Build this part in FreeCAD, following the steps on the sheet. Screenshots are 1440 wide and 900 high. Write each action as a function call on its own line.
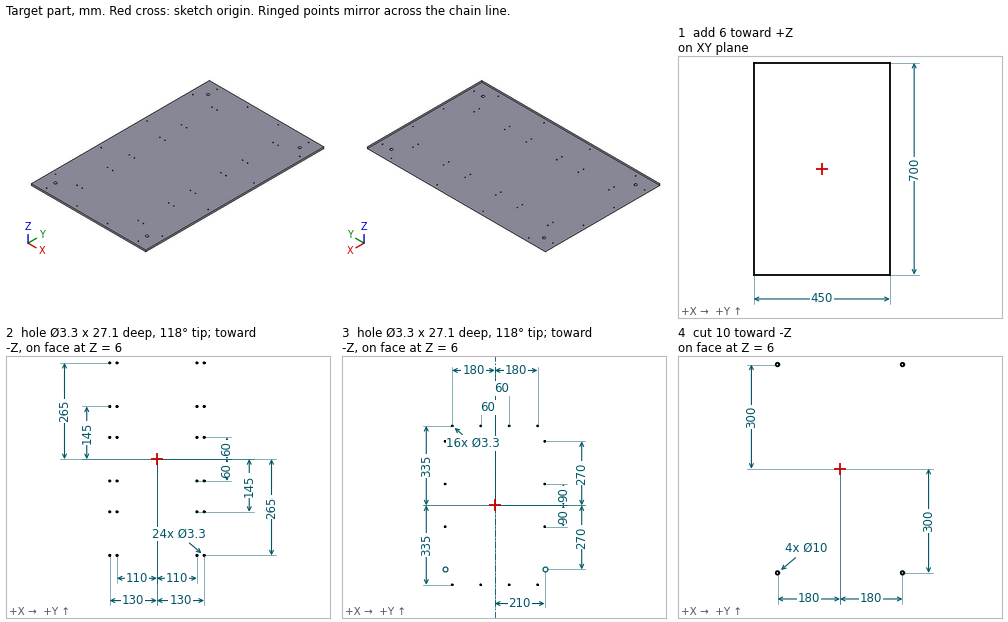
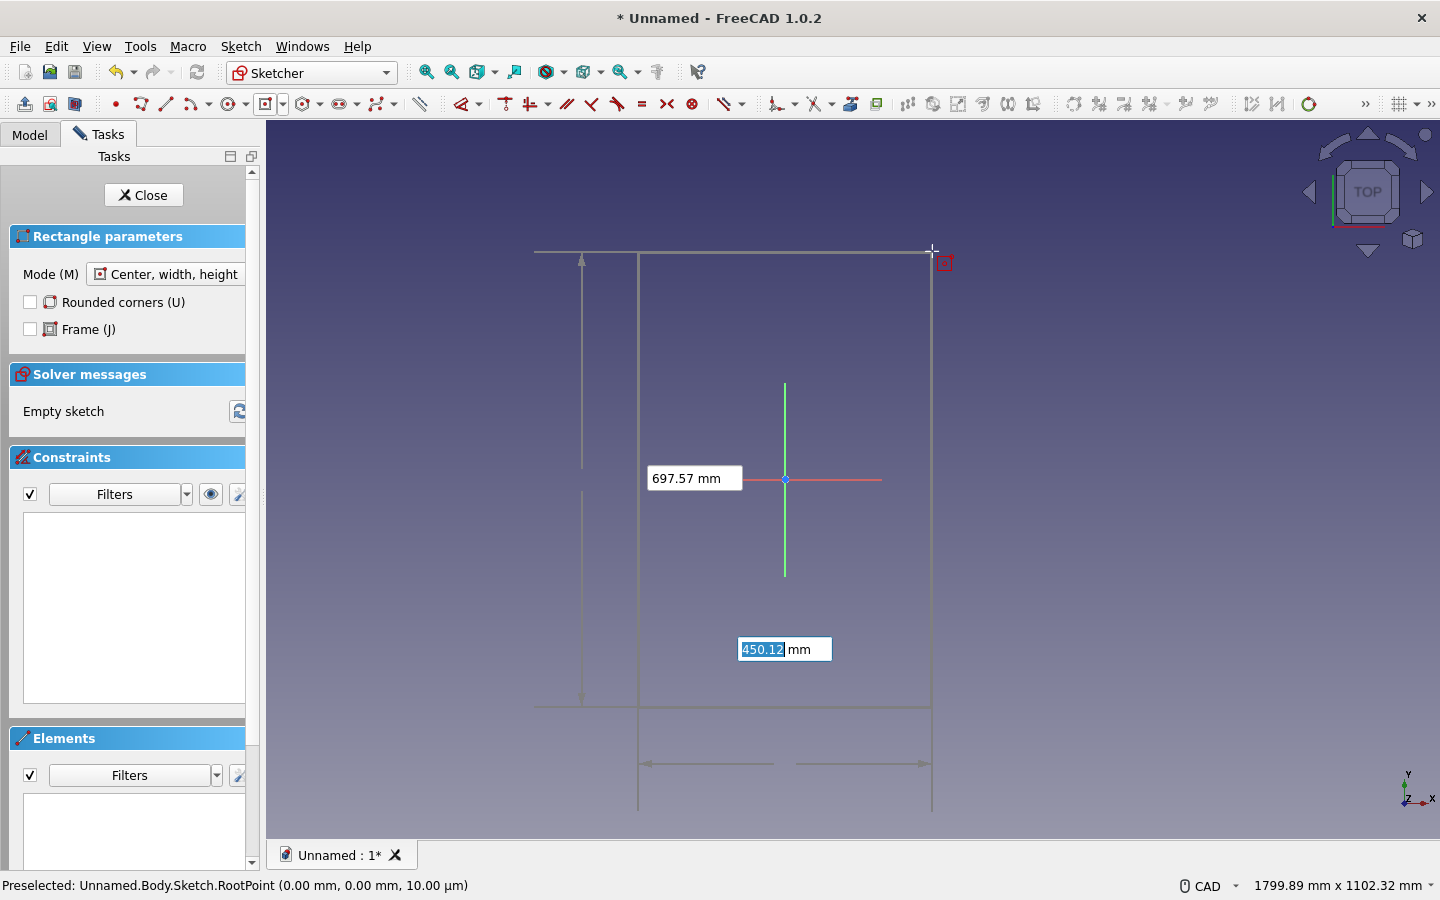
text(450)
key(Tab)
text(700)
key(Return)
key(Escape)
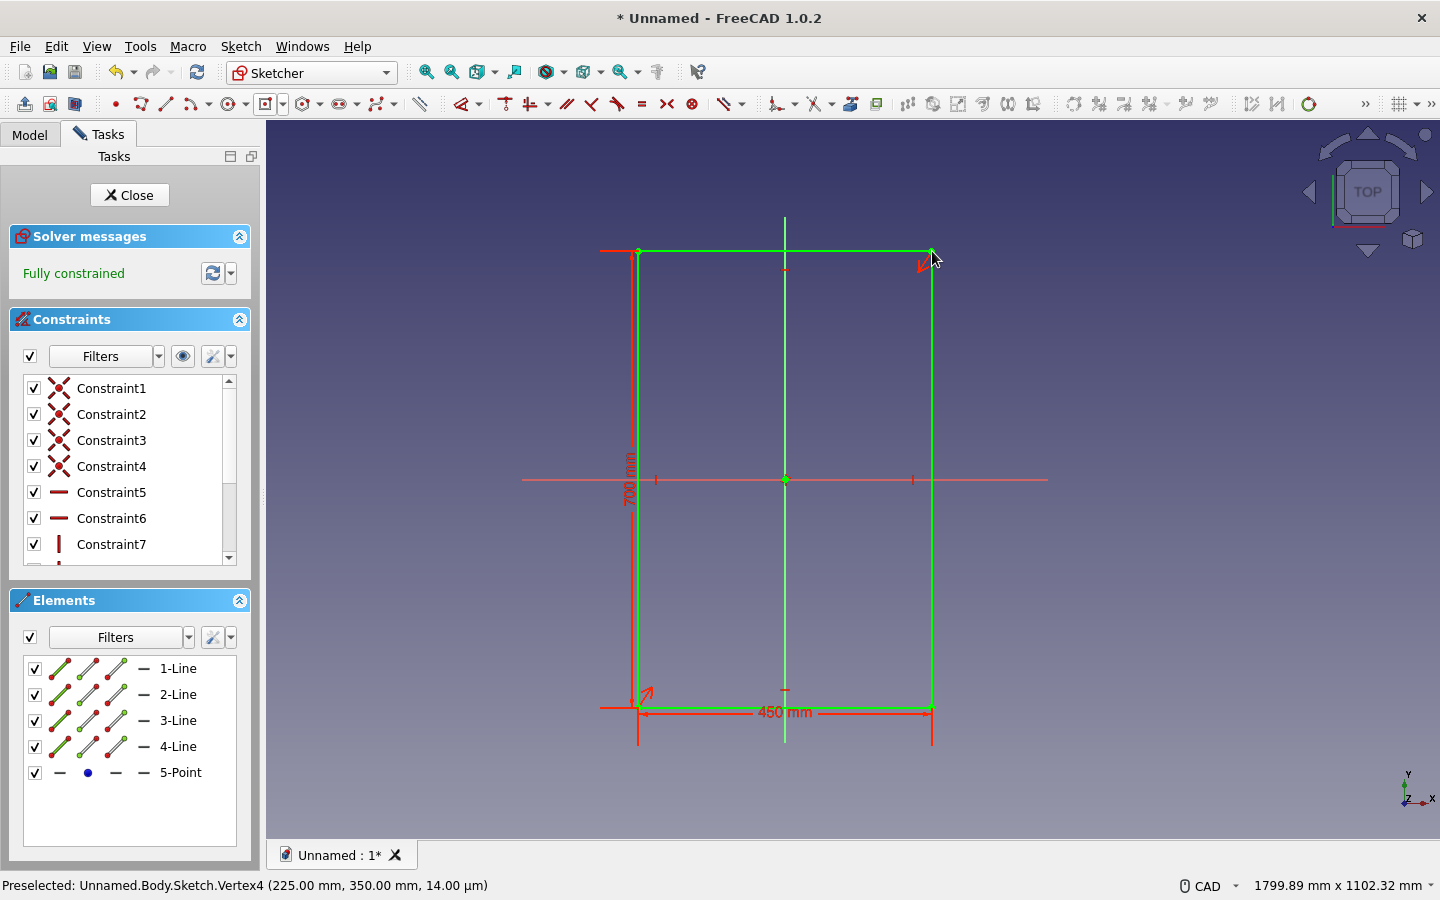
click(130, 195)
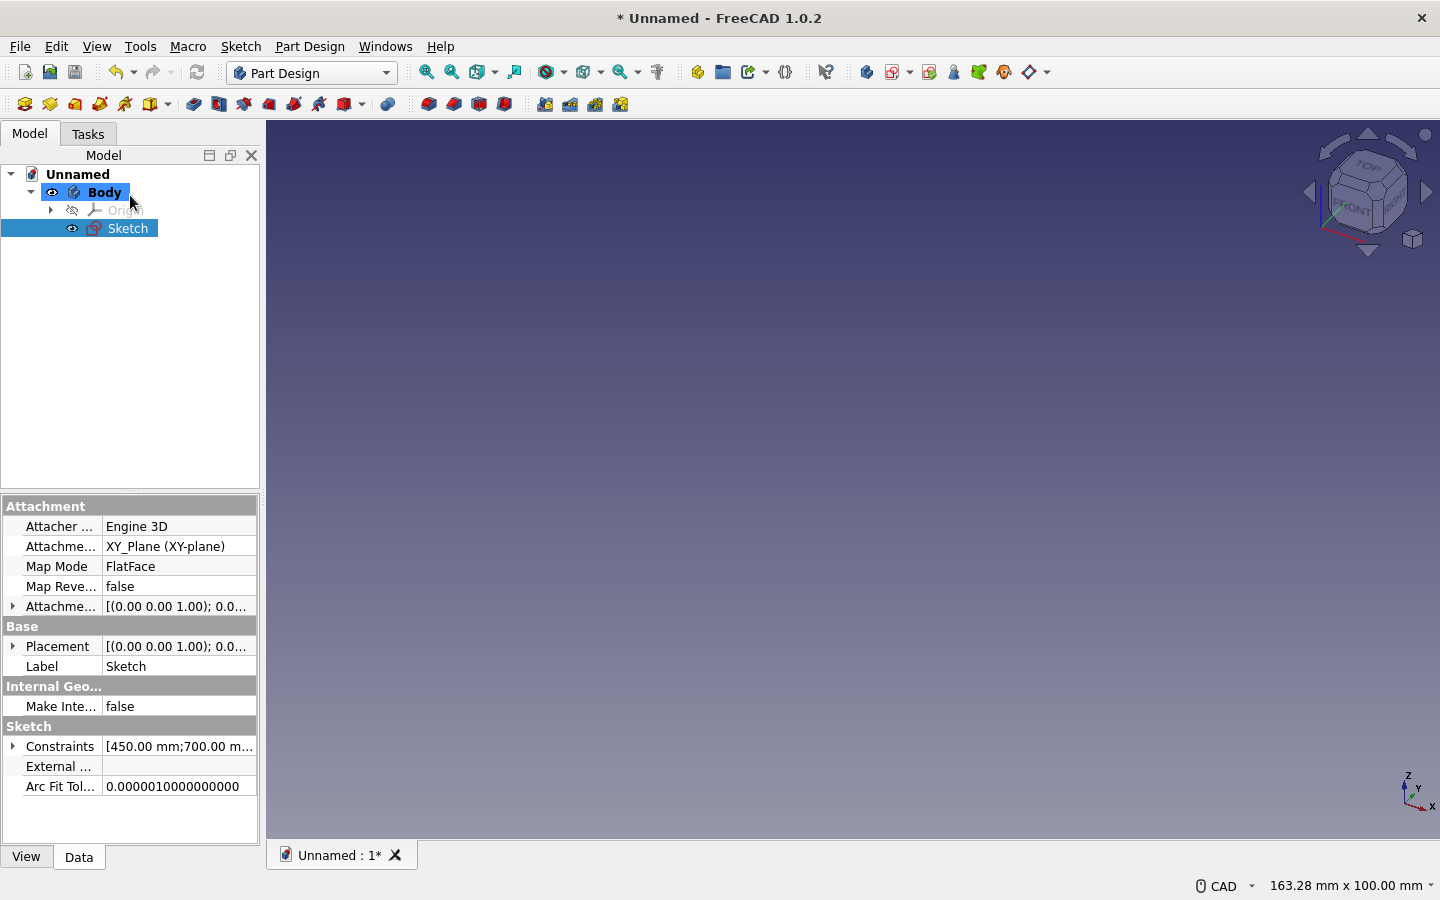
click(25, 104)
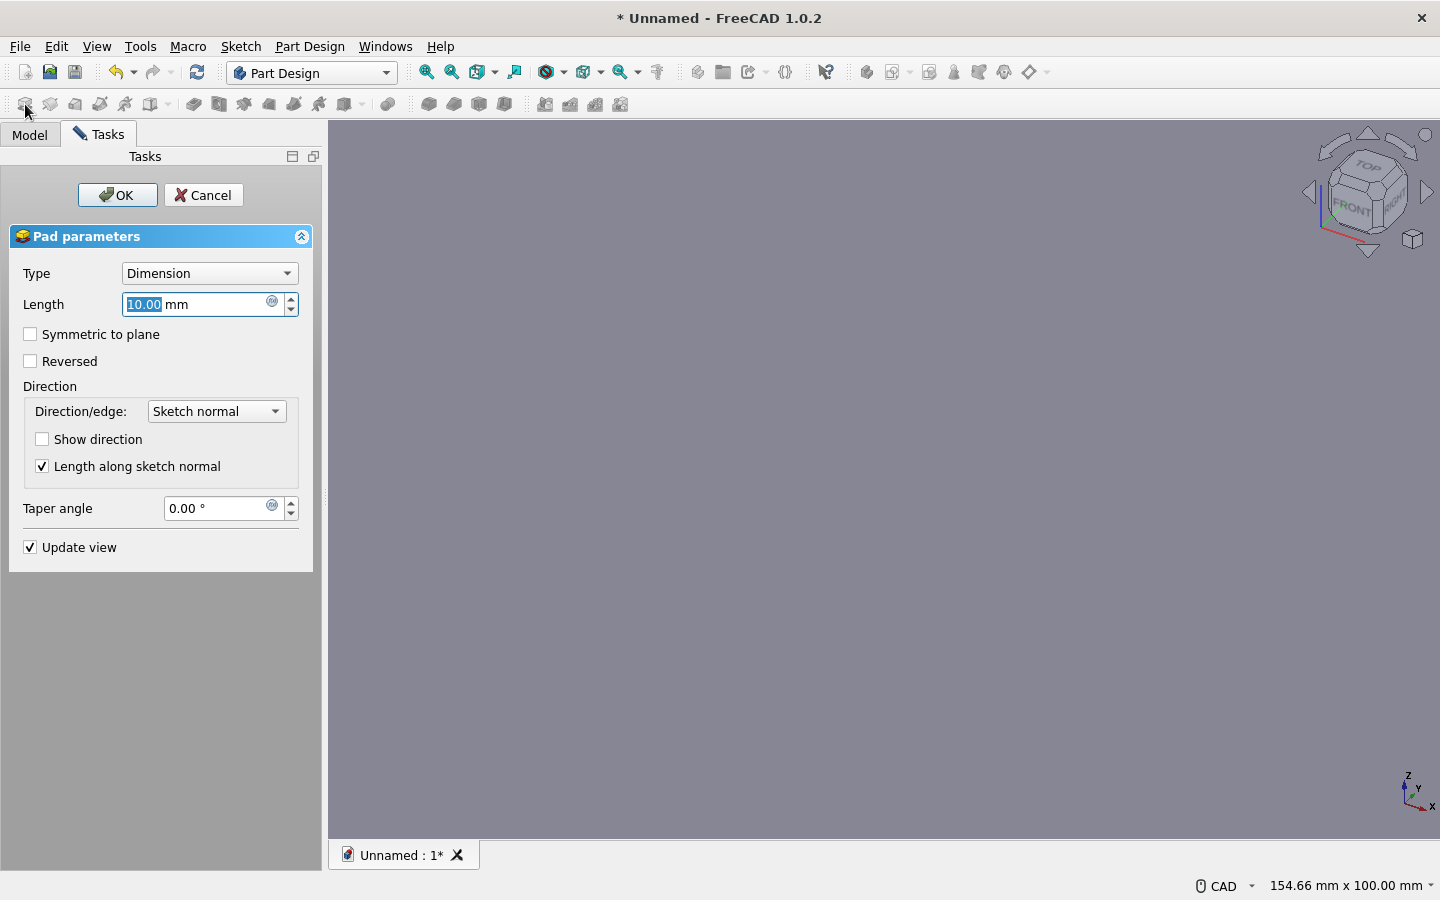
text(6)
key(Tab)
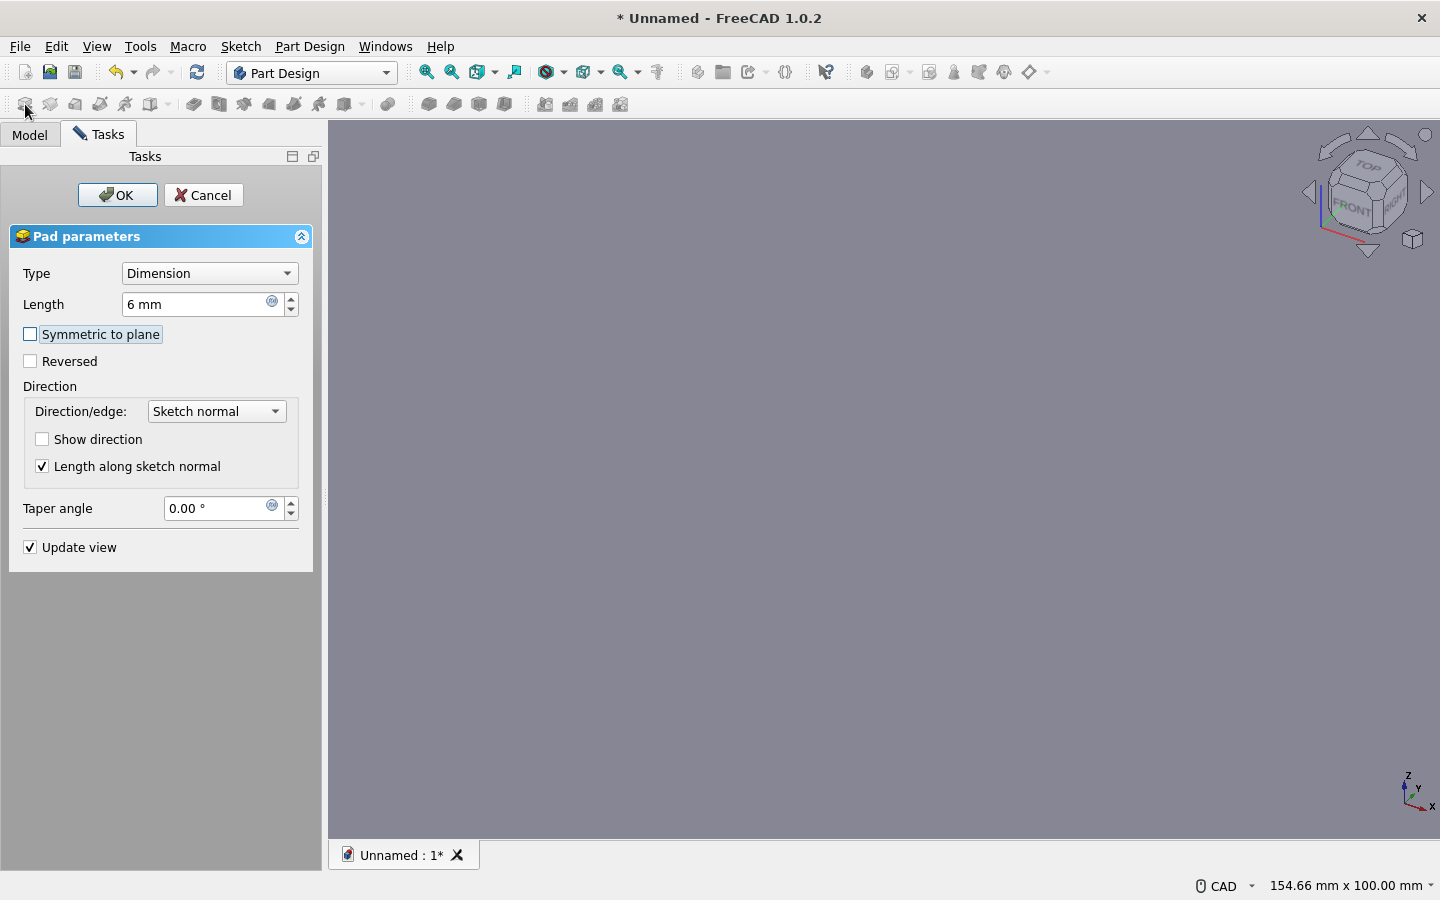
click(118, 195)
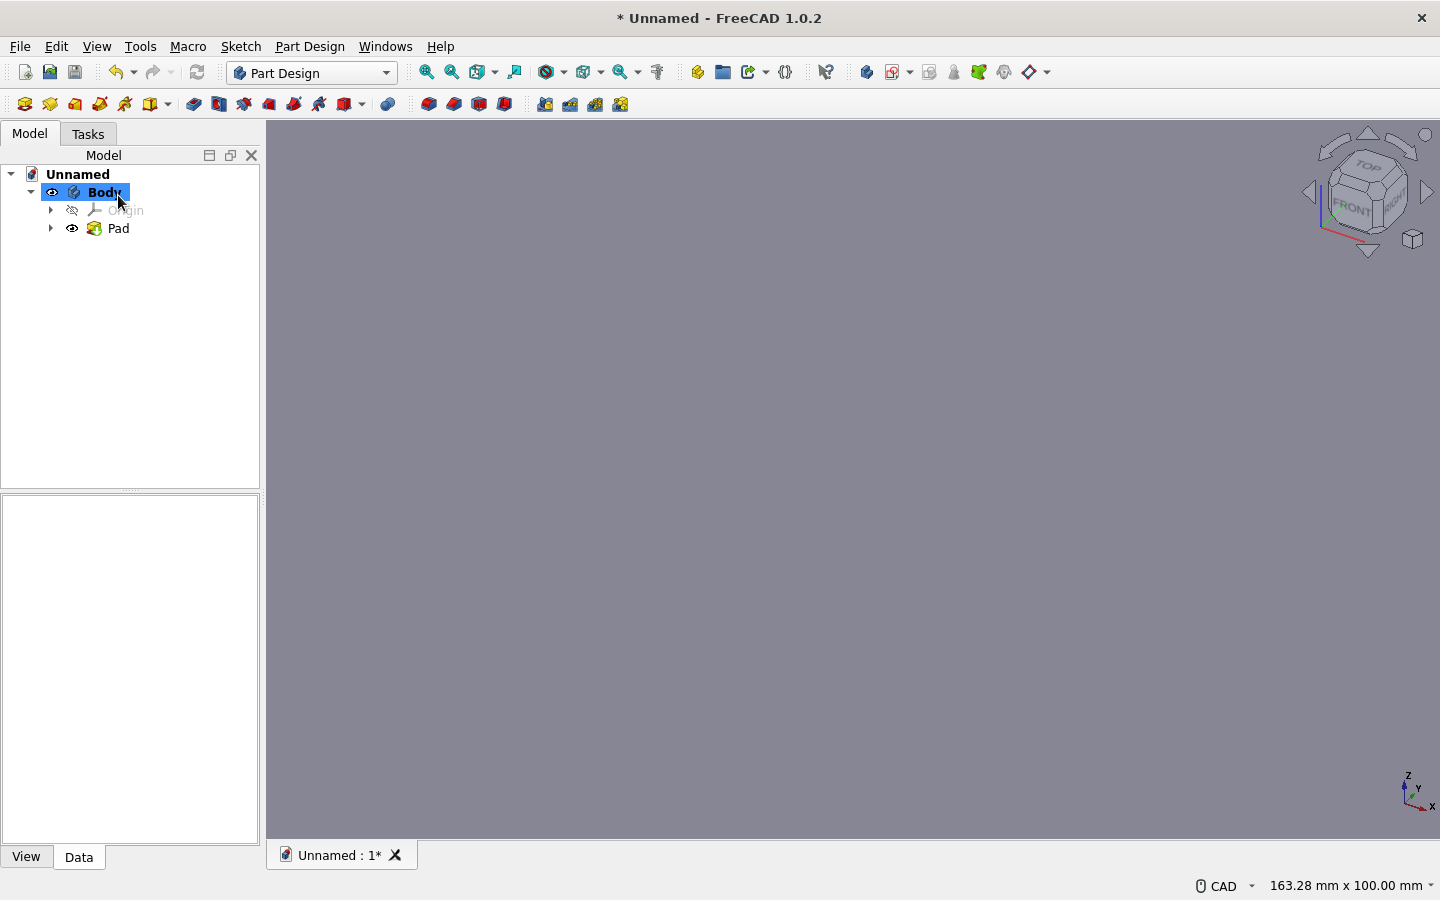
click(427, 72)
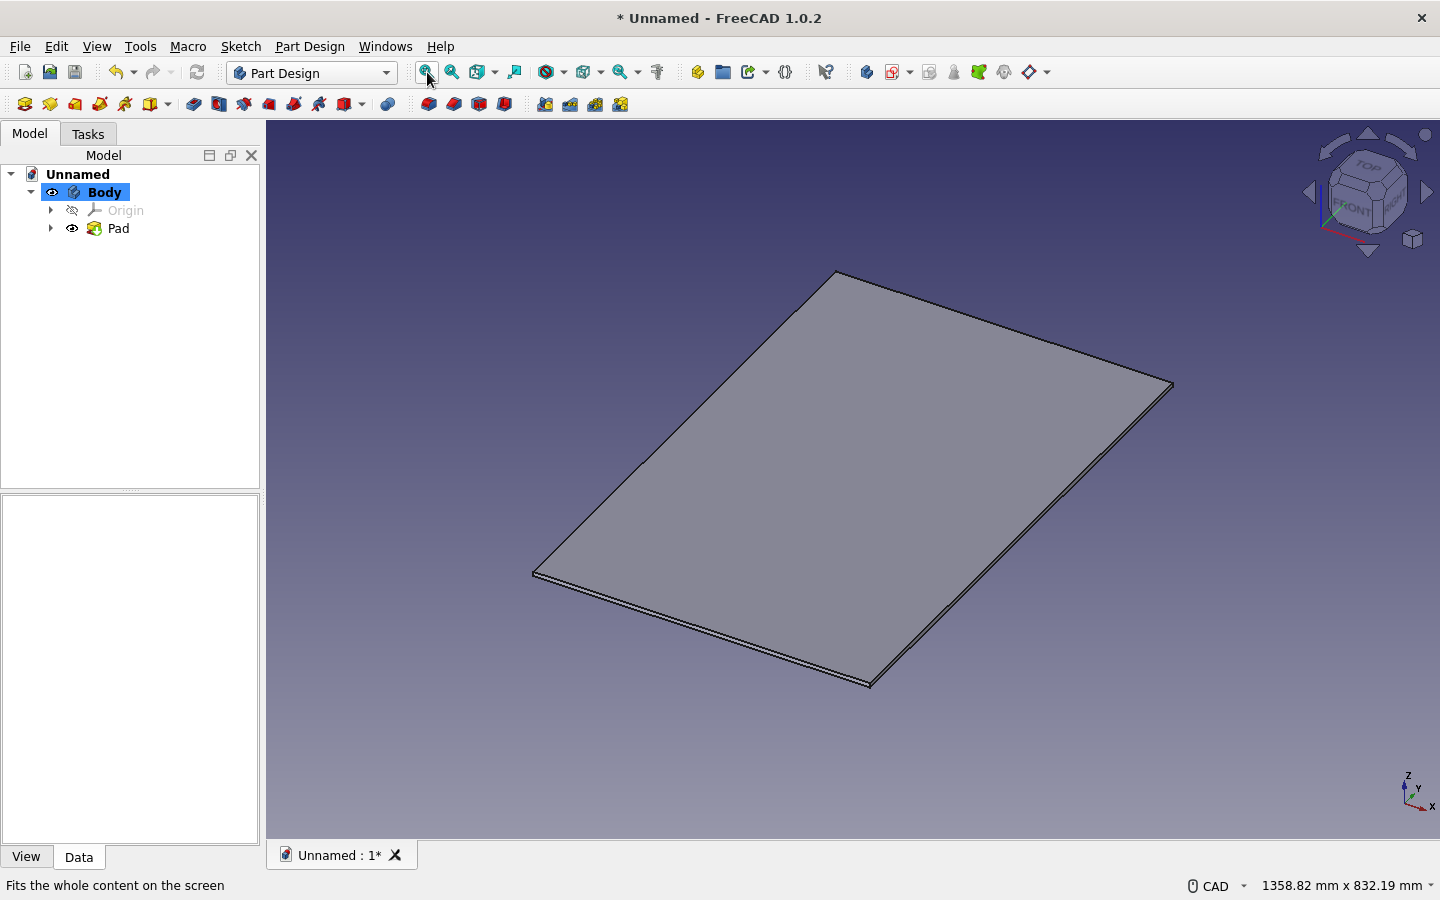
click(896, 433)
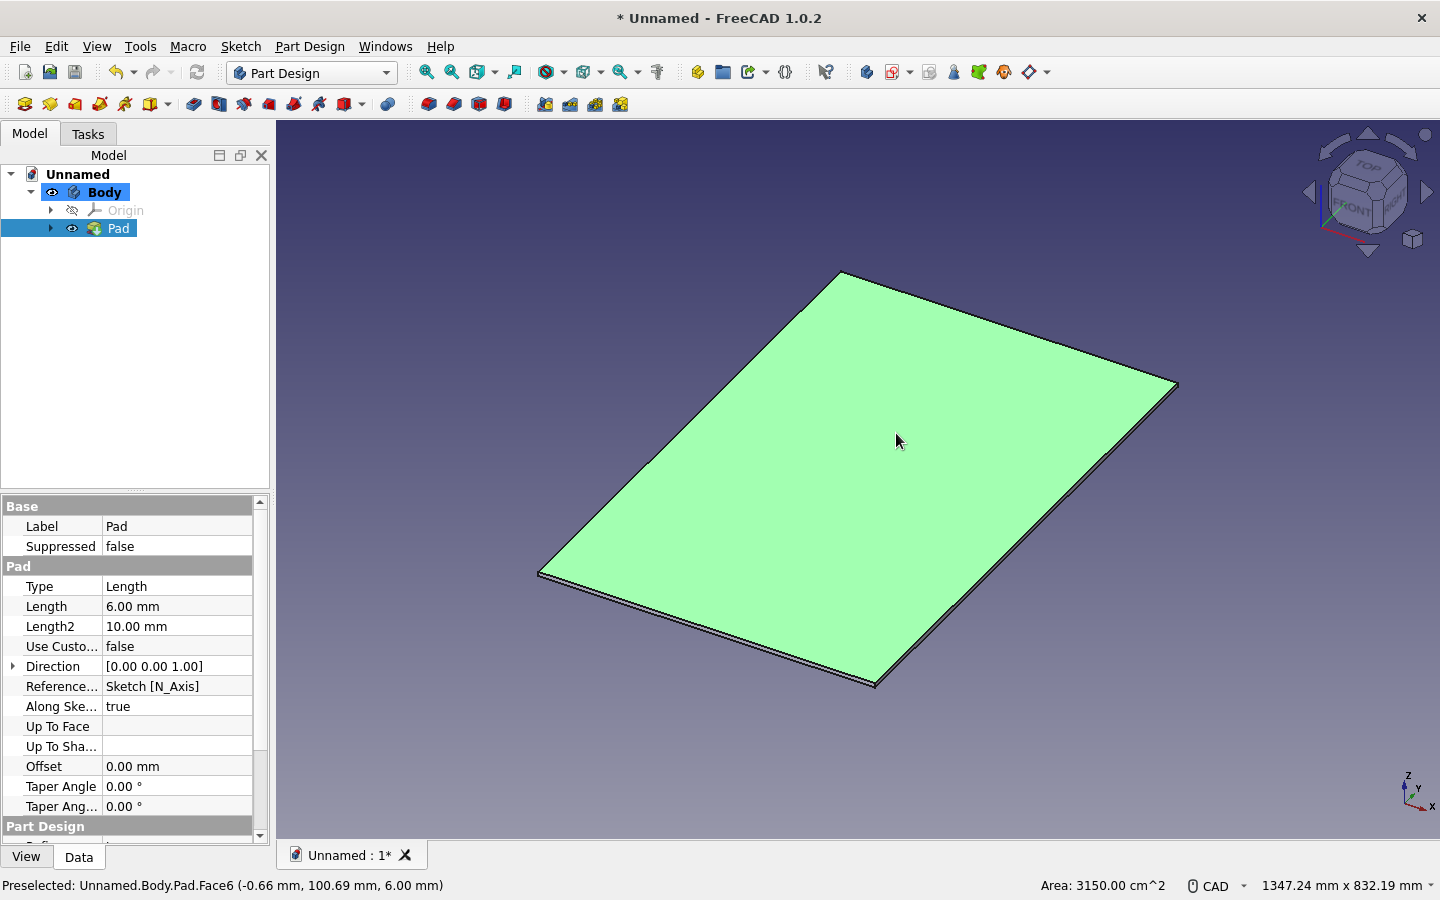
click(892, 72)